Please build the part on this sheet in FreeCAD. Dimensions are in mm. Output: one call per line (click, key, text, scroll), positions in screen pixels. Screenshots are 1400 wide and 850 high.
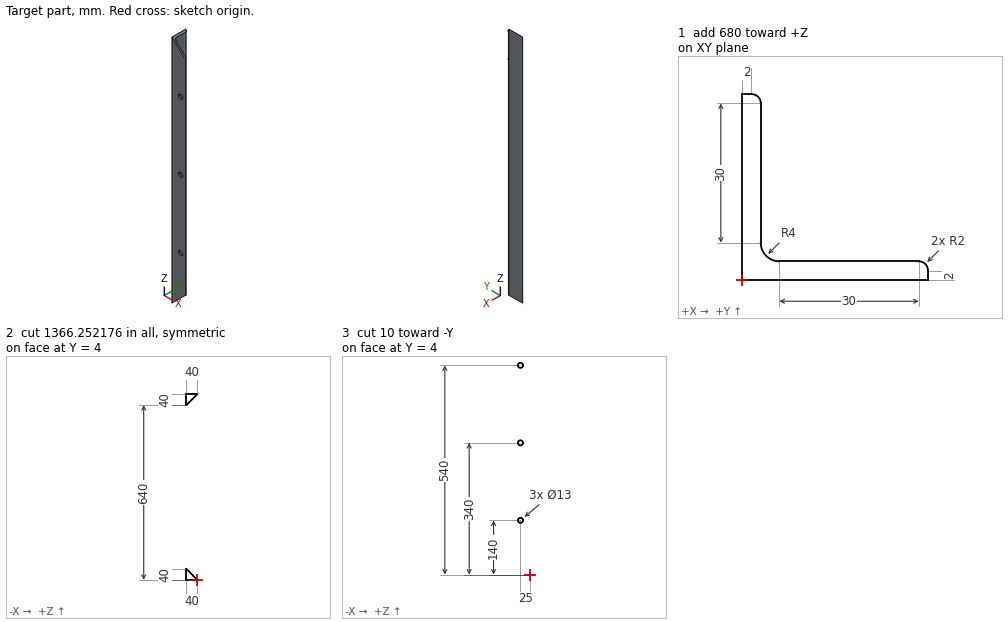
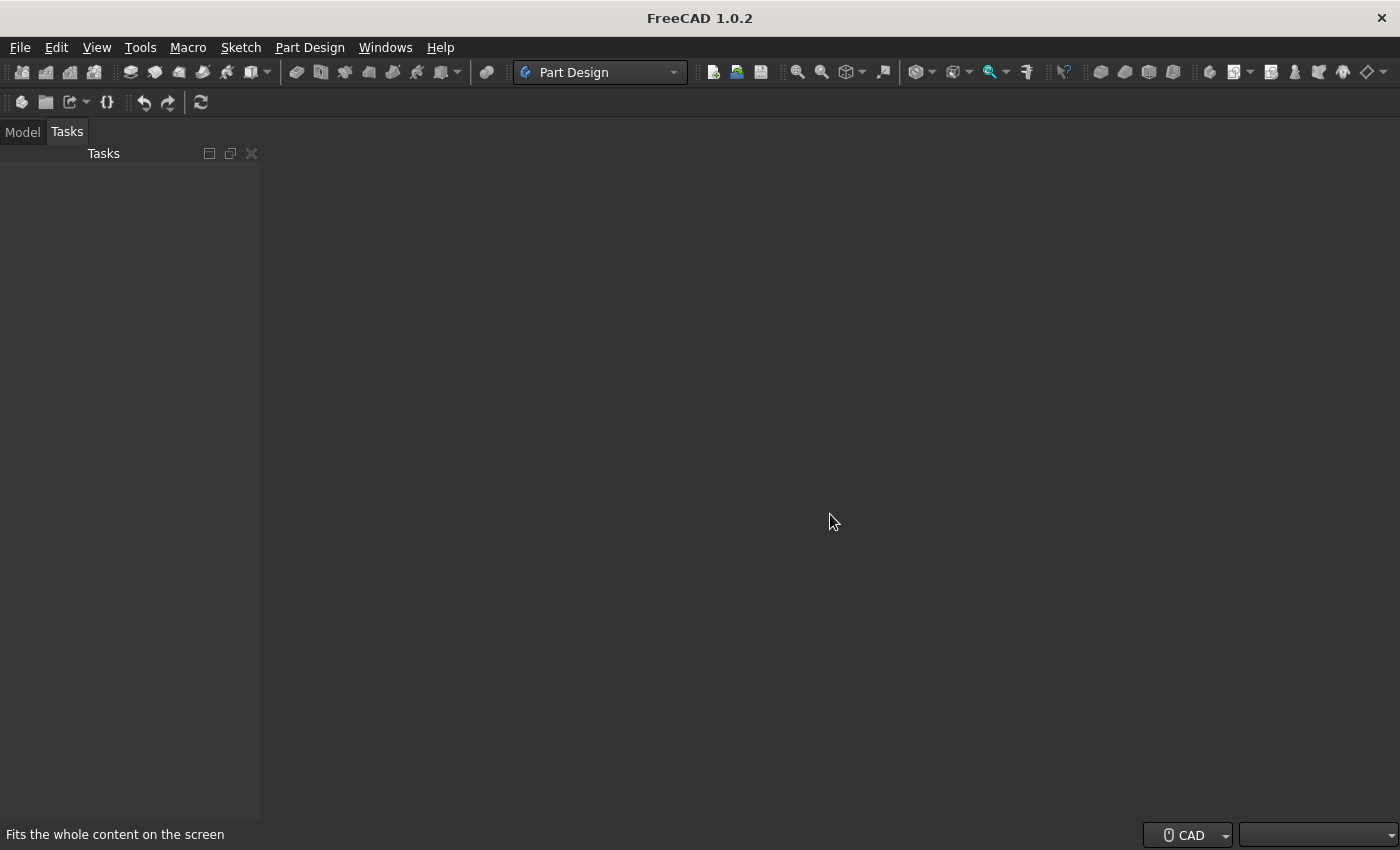
click(714, 72)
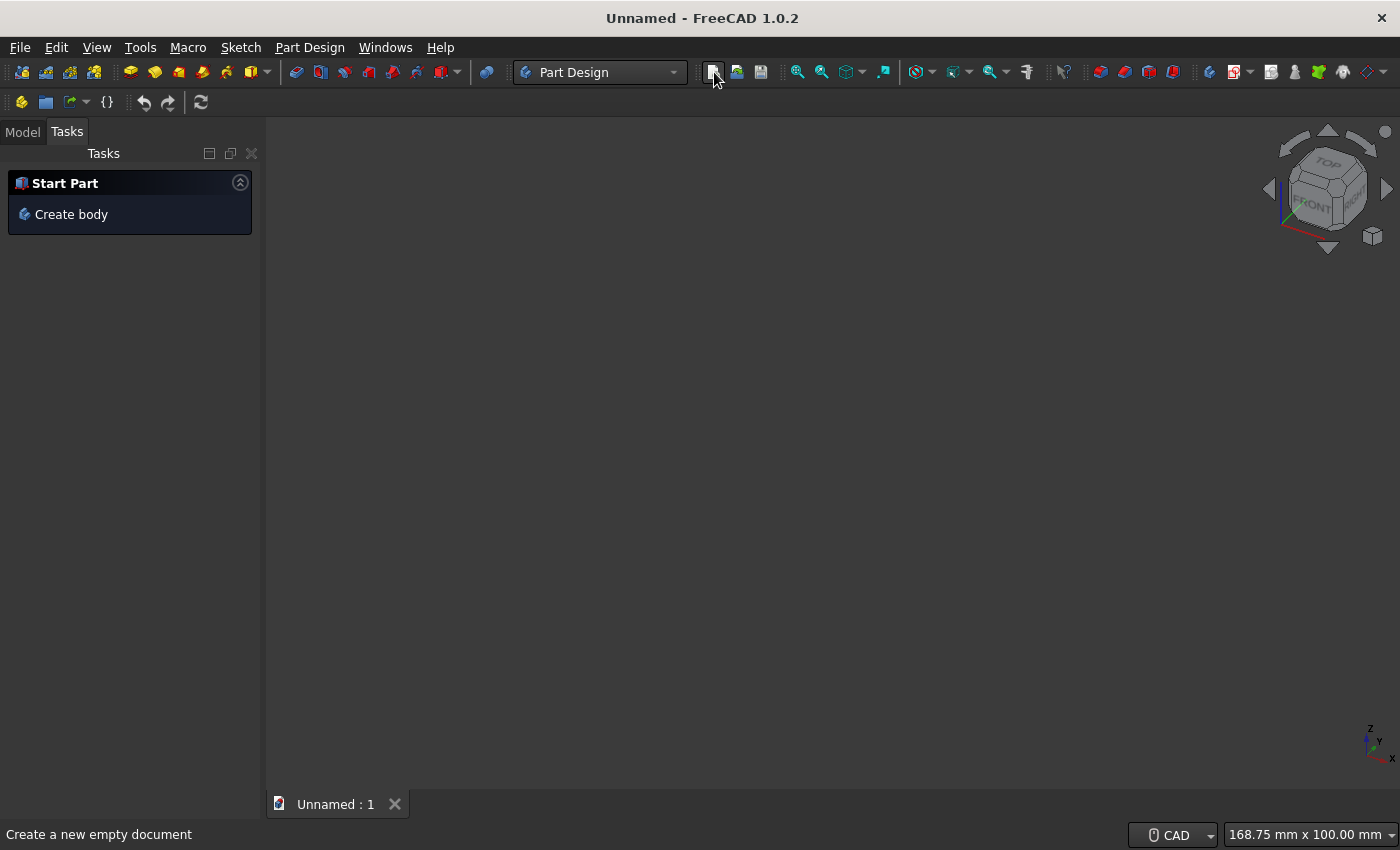
click(1234, 72)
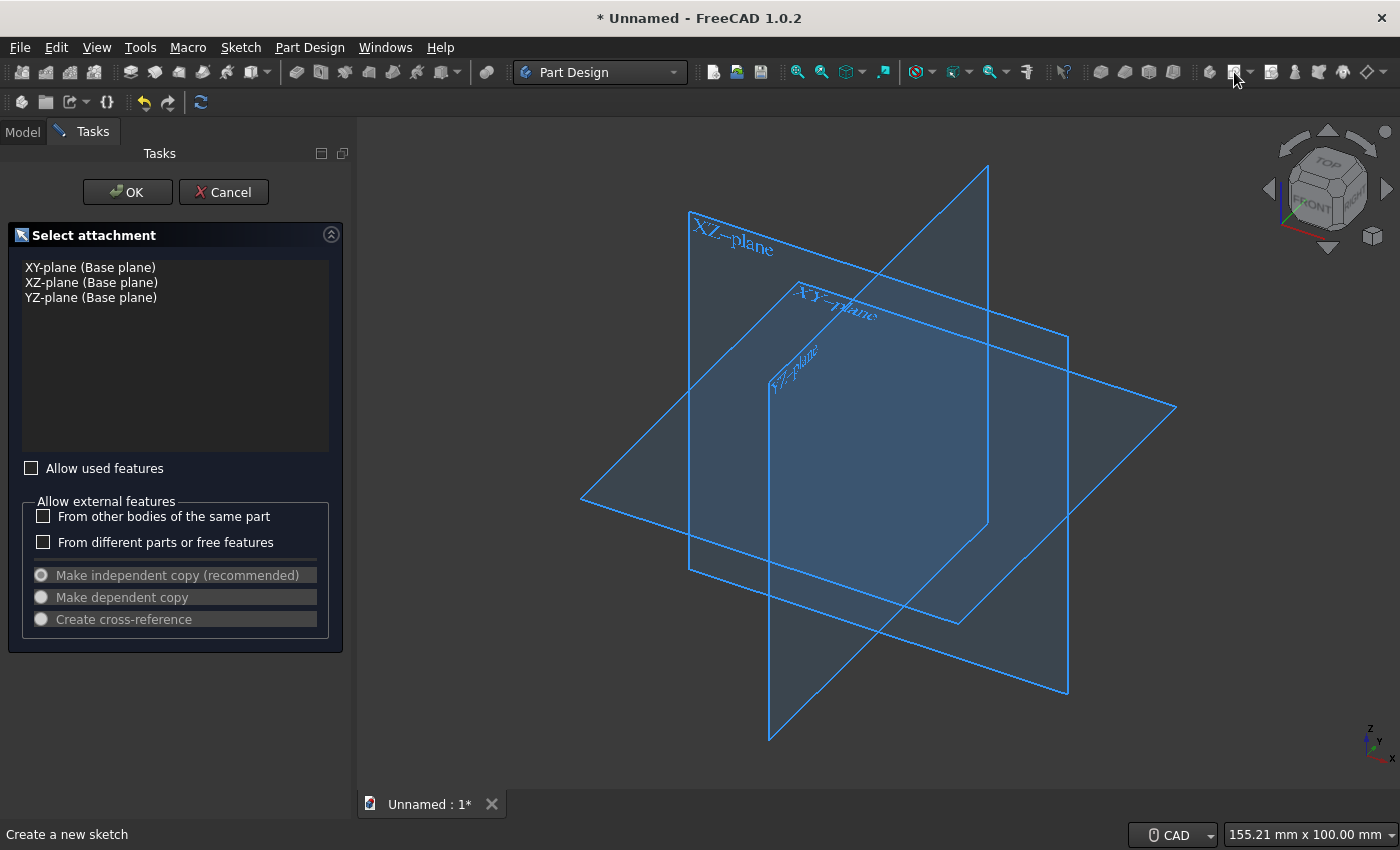
click(82, 268)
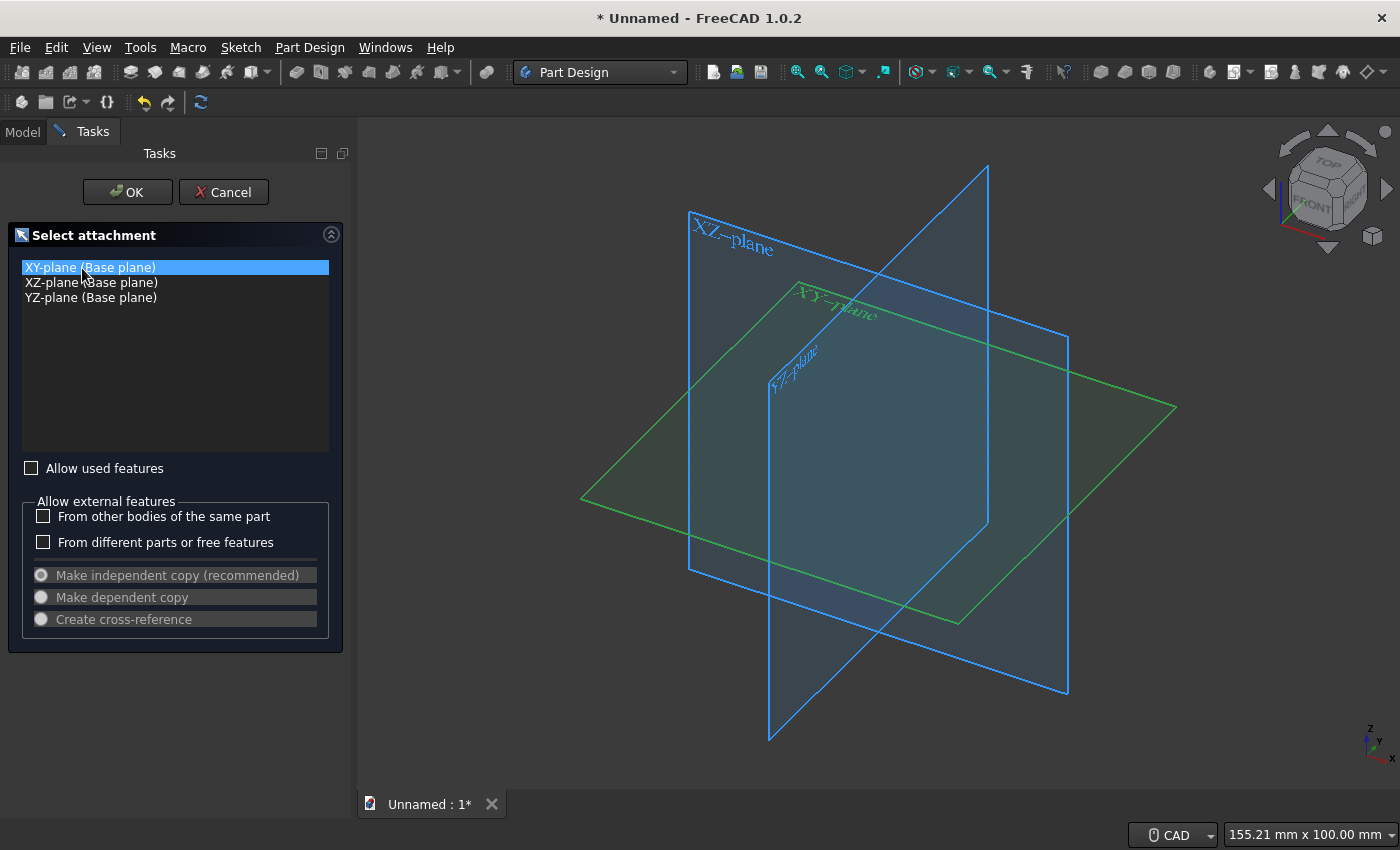
click(128, 192)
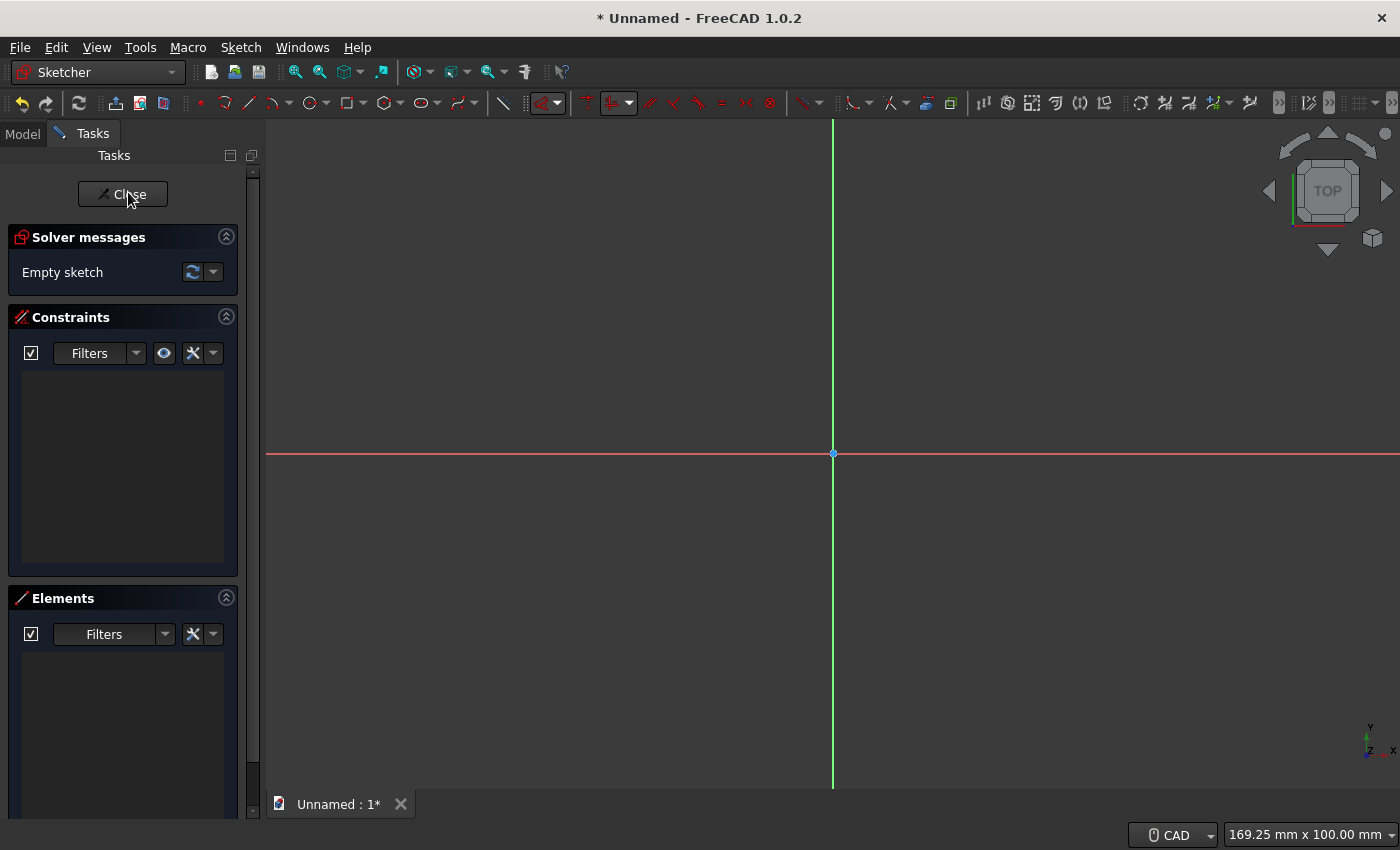
scroll(1235, 147, up, 2)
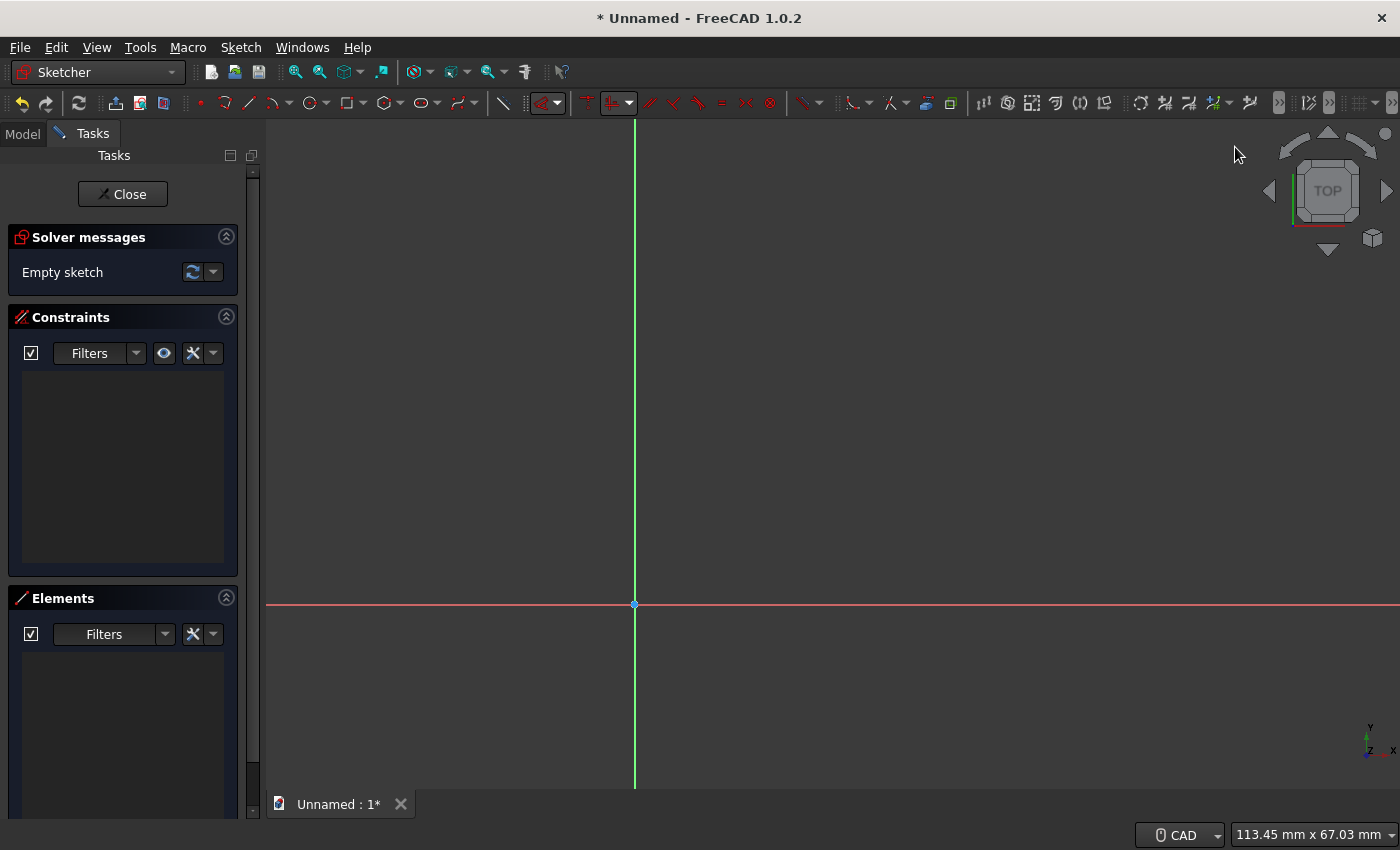
click(250, 104)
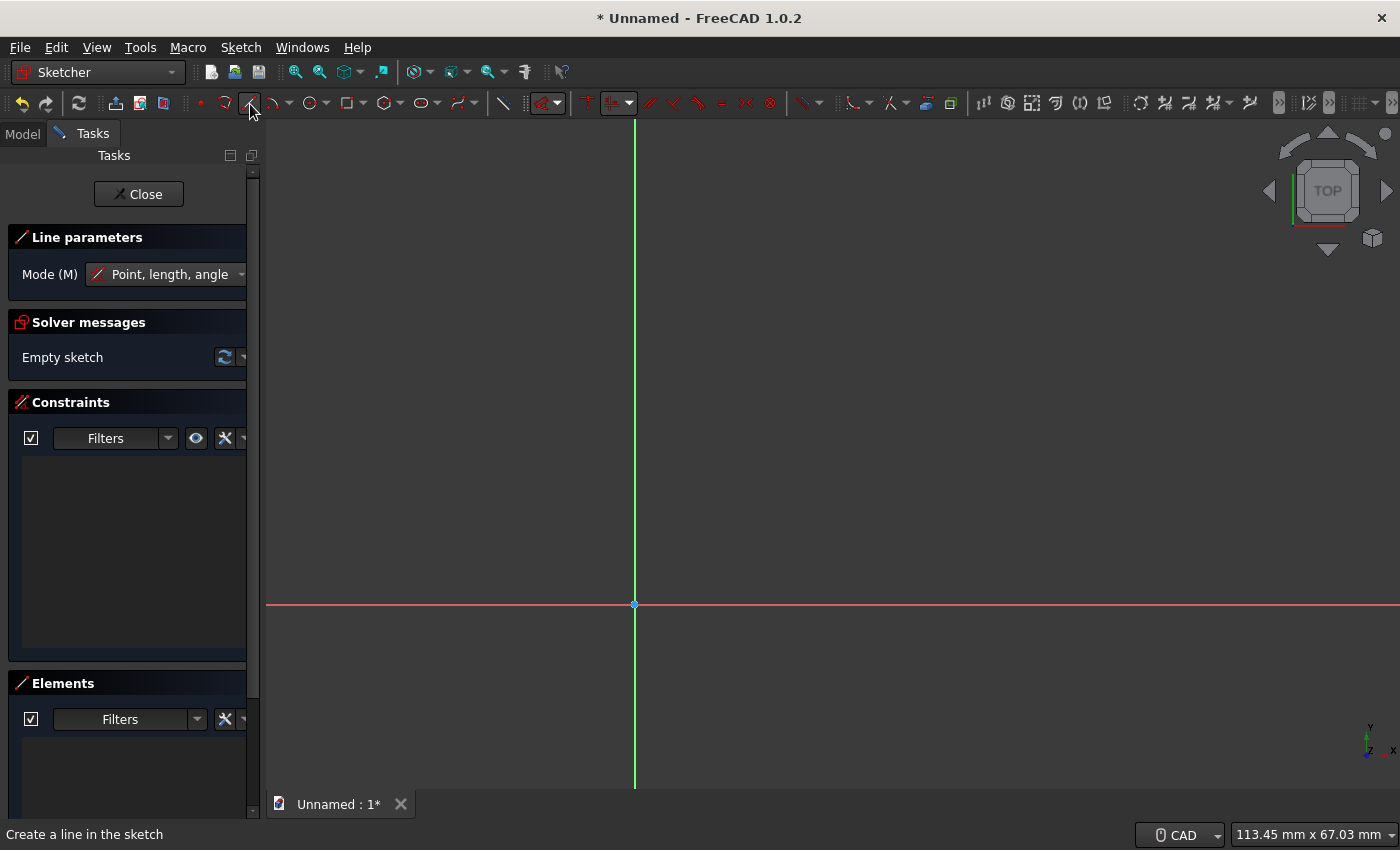
click(1015, 565)
click(715, 565)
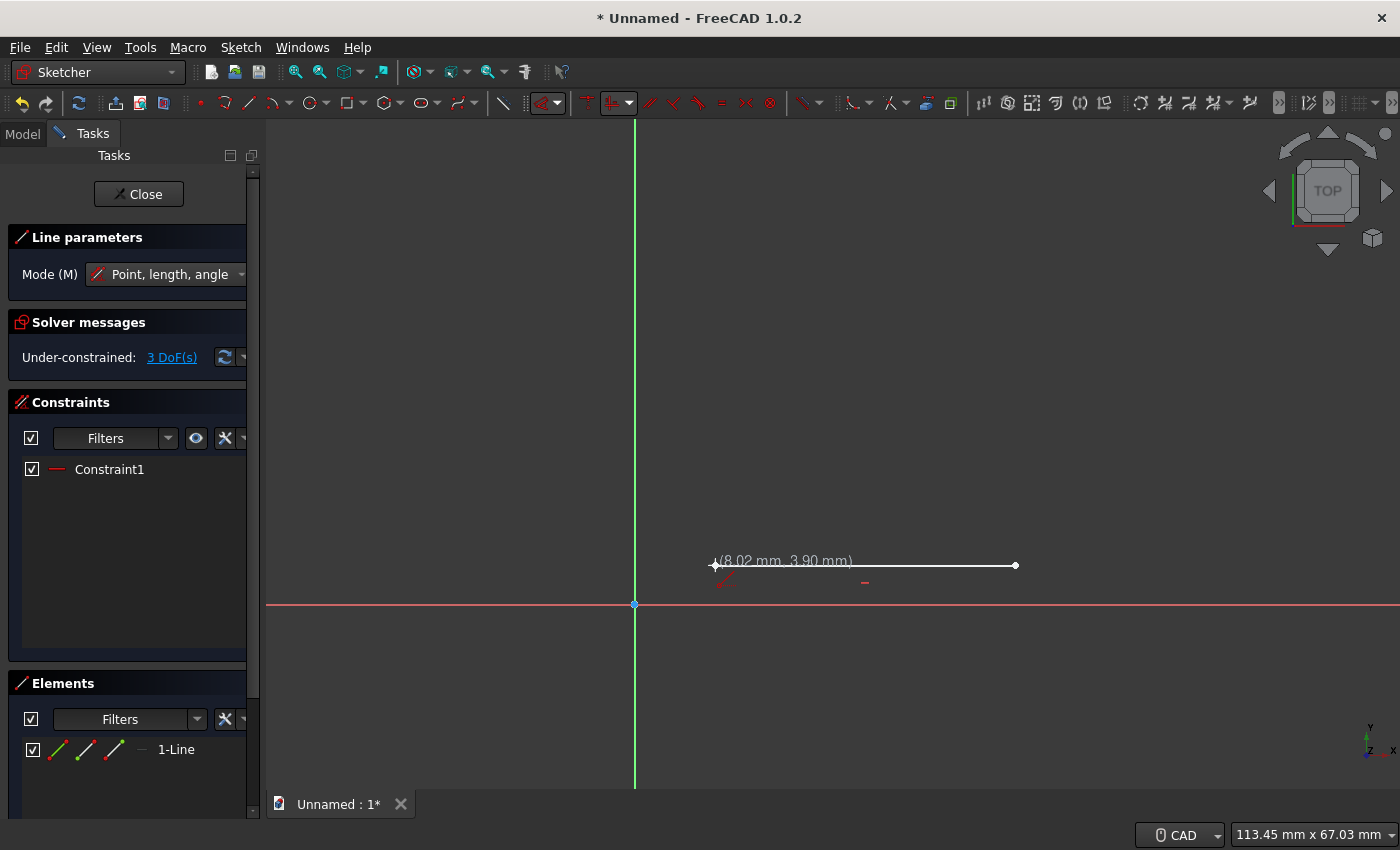
click(675, 525)
click(675, 225)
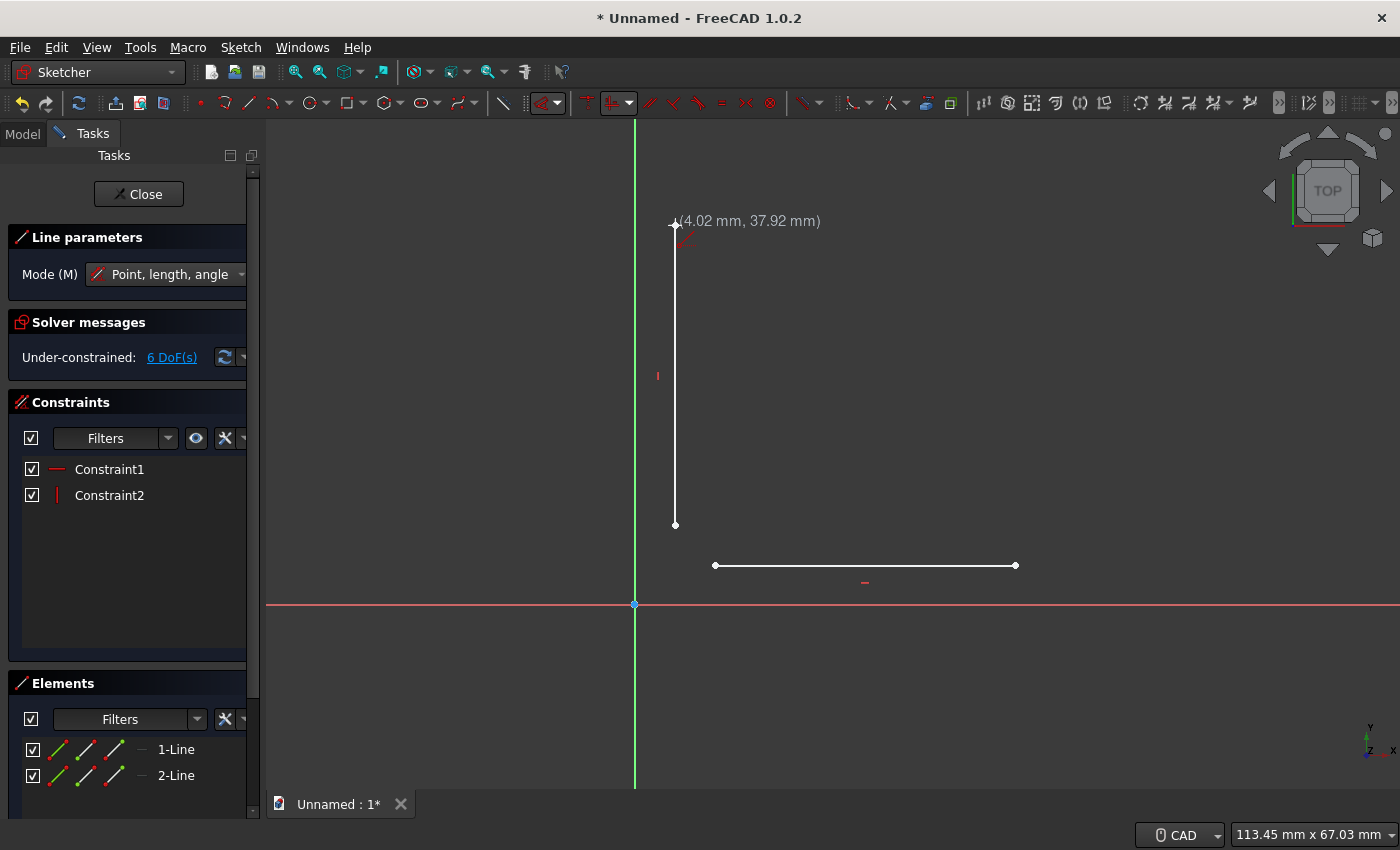
click(226, 104)